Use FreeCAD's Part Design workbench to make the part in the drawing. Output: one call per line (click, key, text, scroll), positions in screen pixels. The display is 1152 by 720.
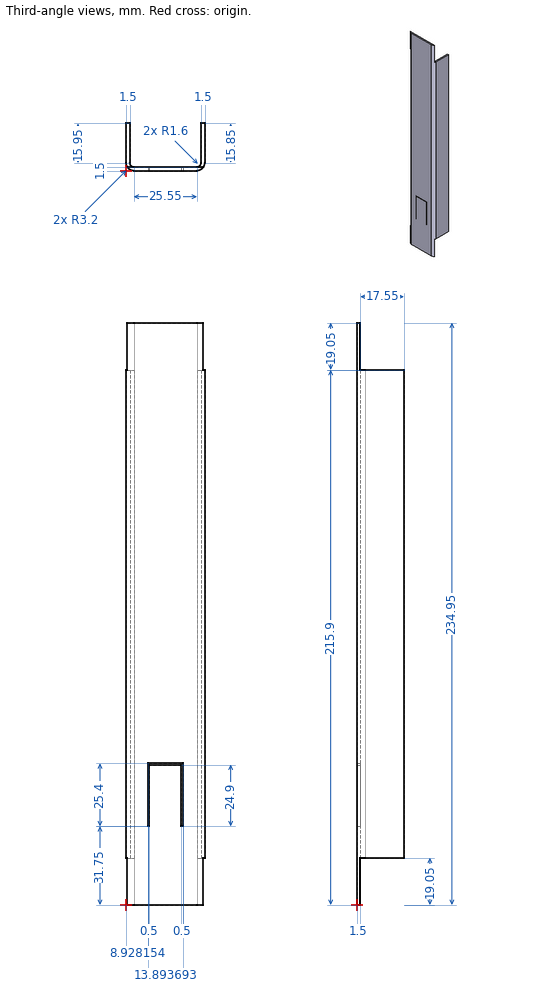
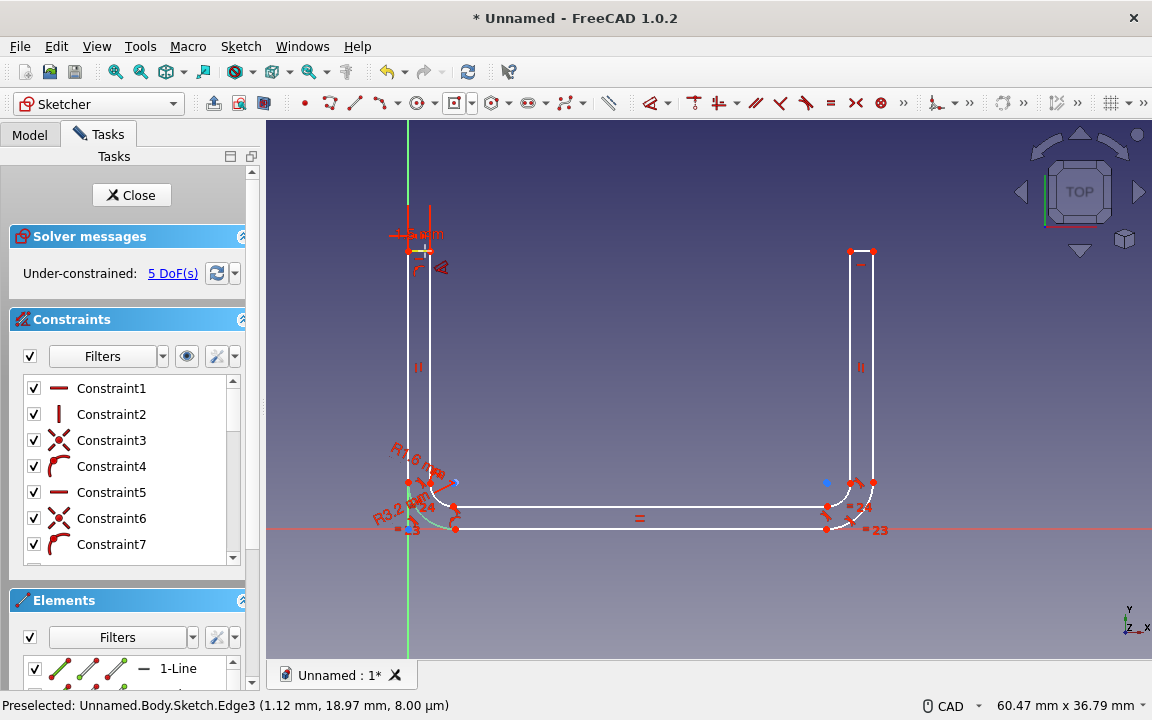
scroll(866, 251, up, 4)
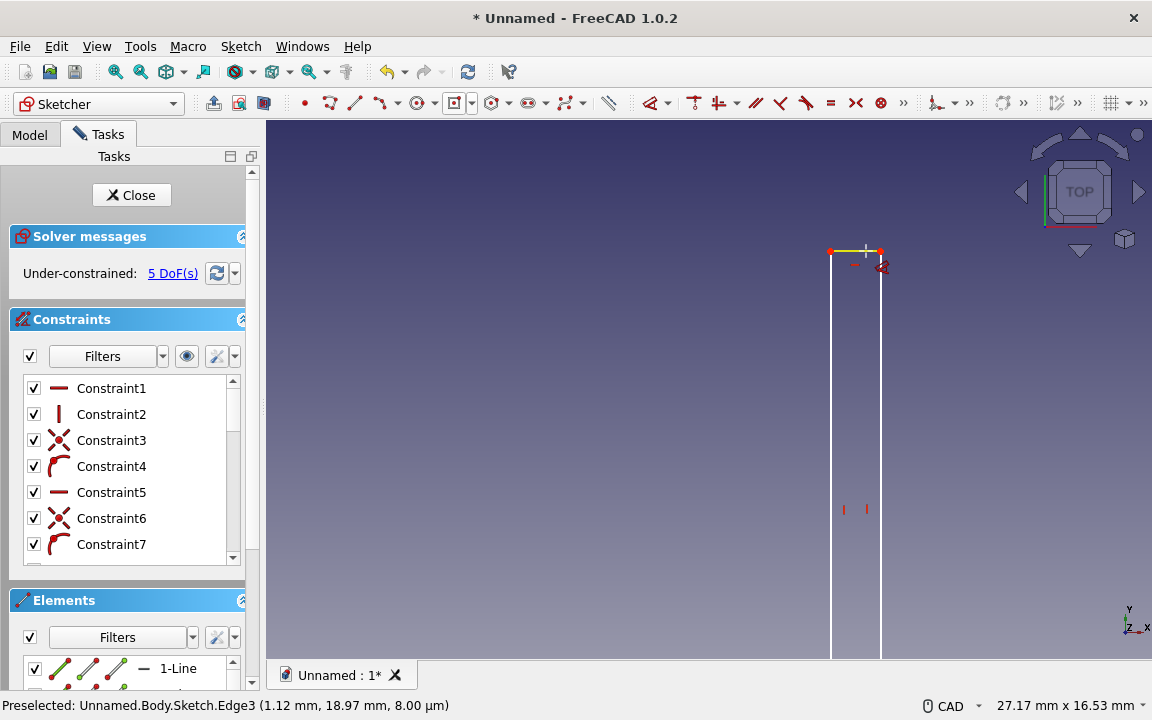
click(866, 251)
click(856, 217)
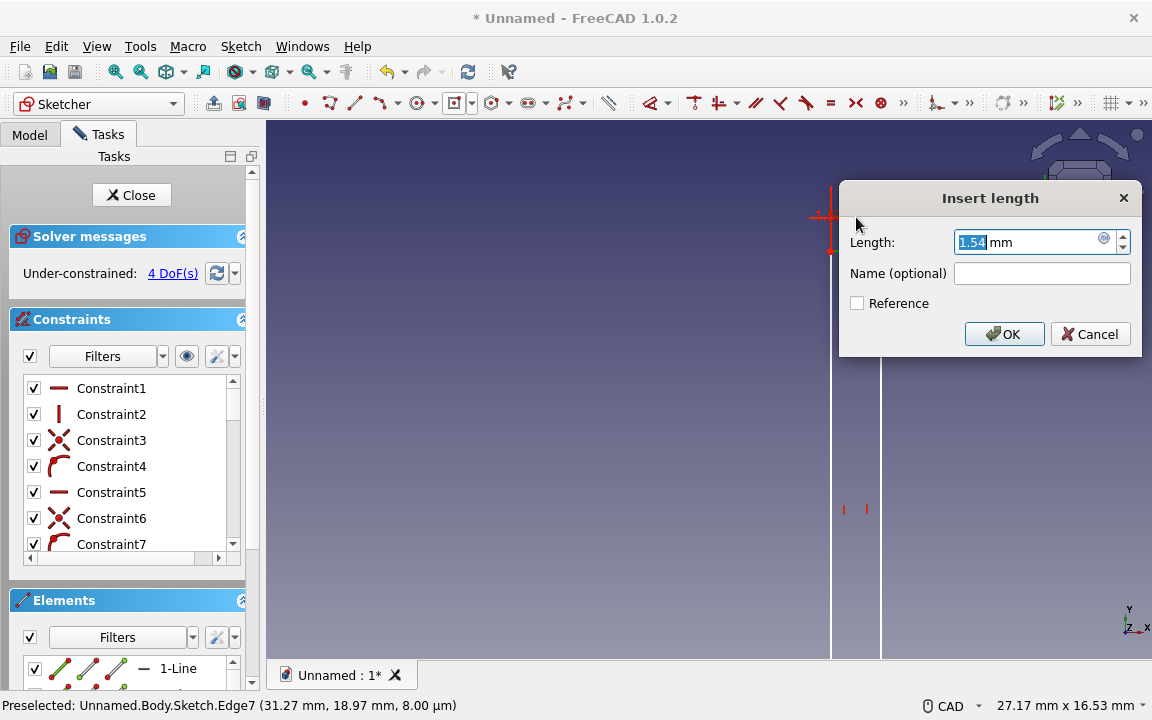
text(1.5)
key(Return)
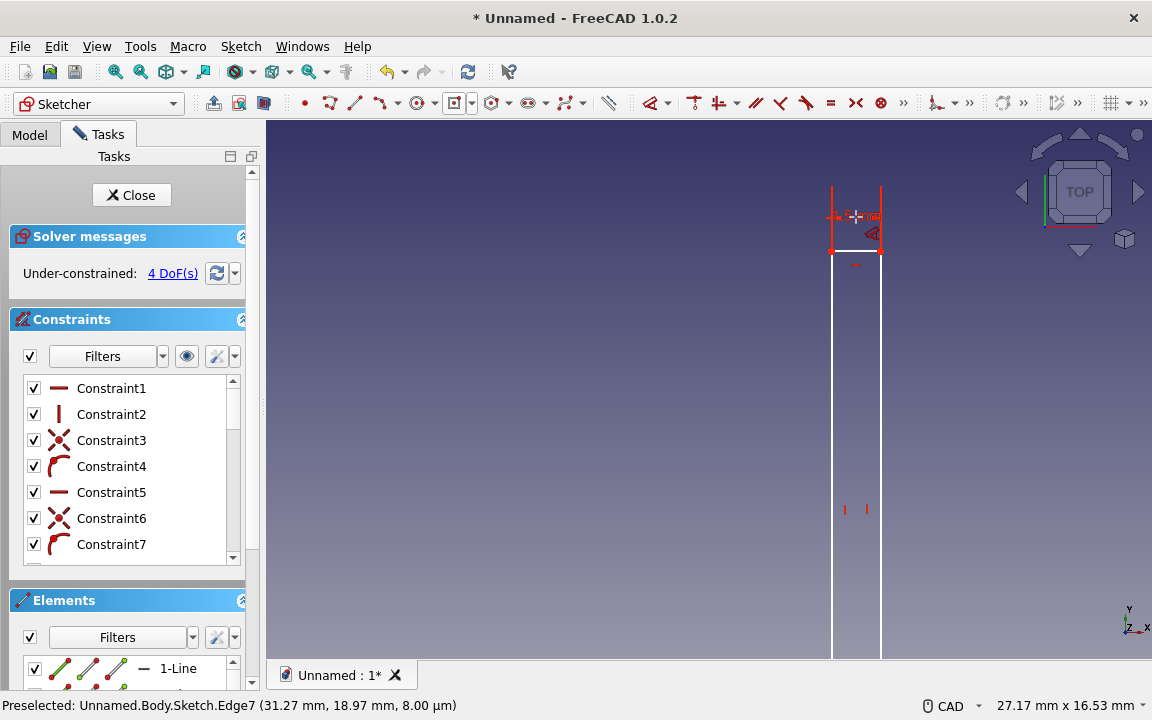
scroll(866, 251, down, 4)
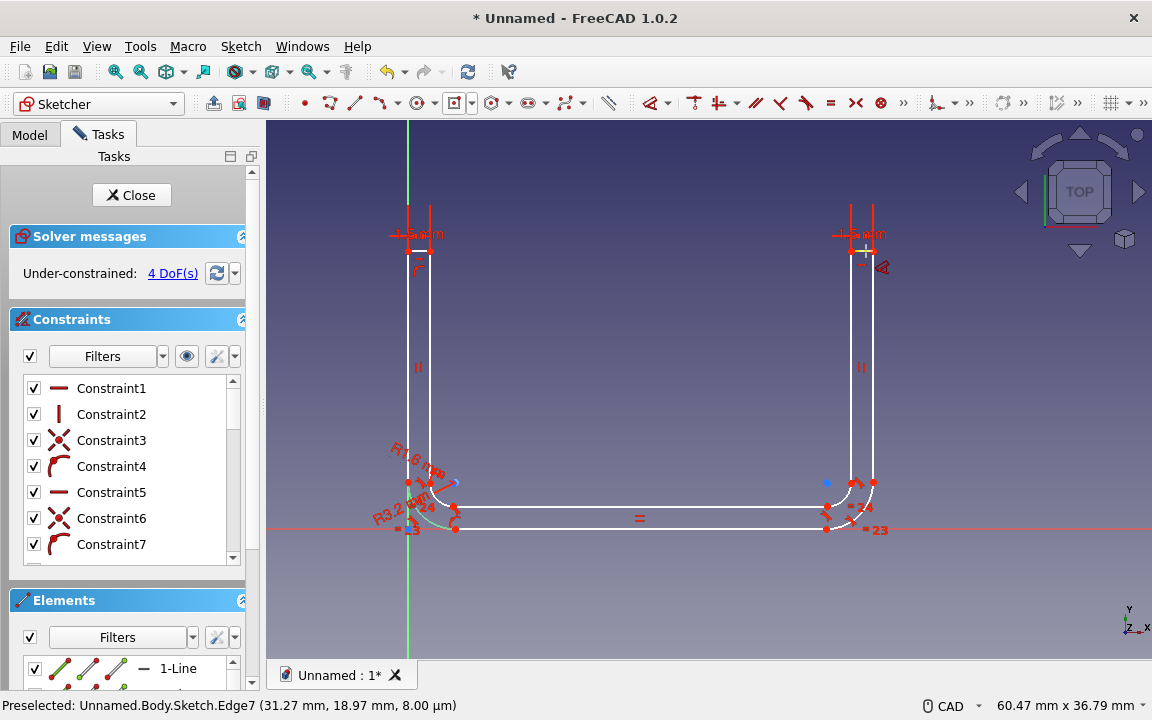
scroll(828, 507, up, 3)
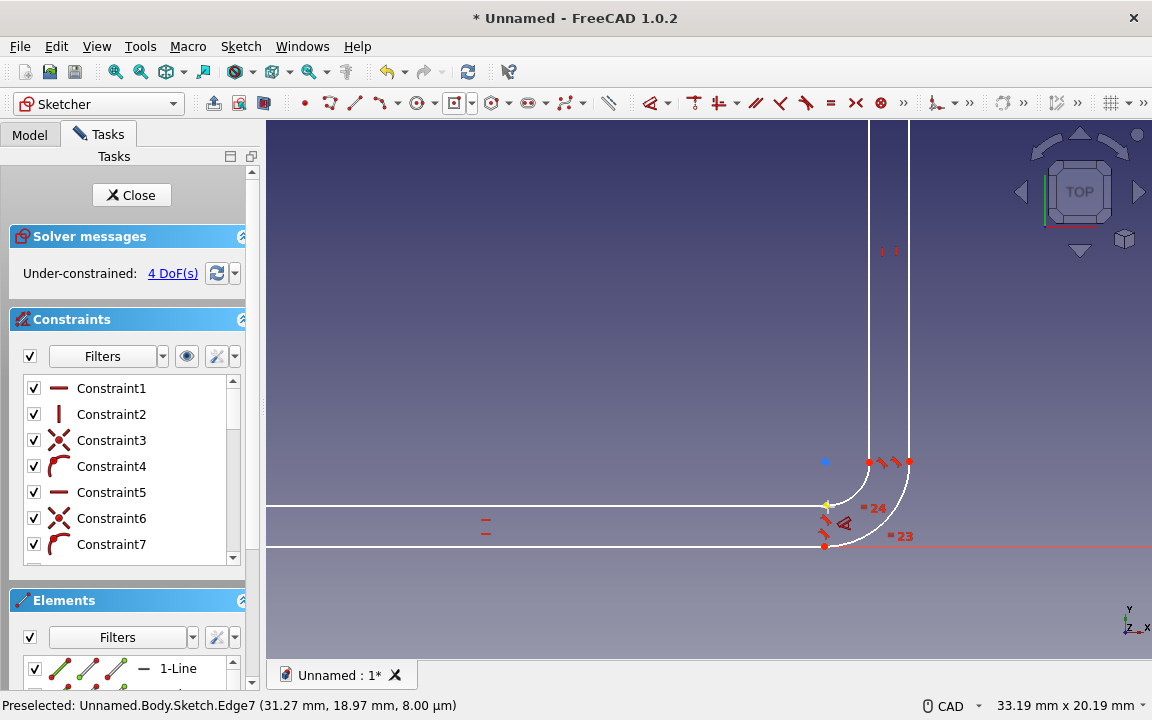
click(827, 506)
click(861, 517)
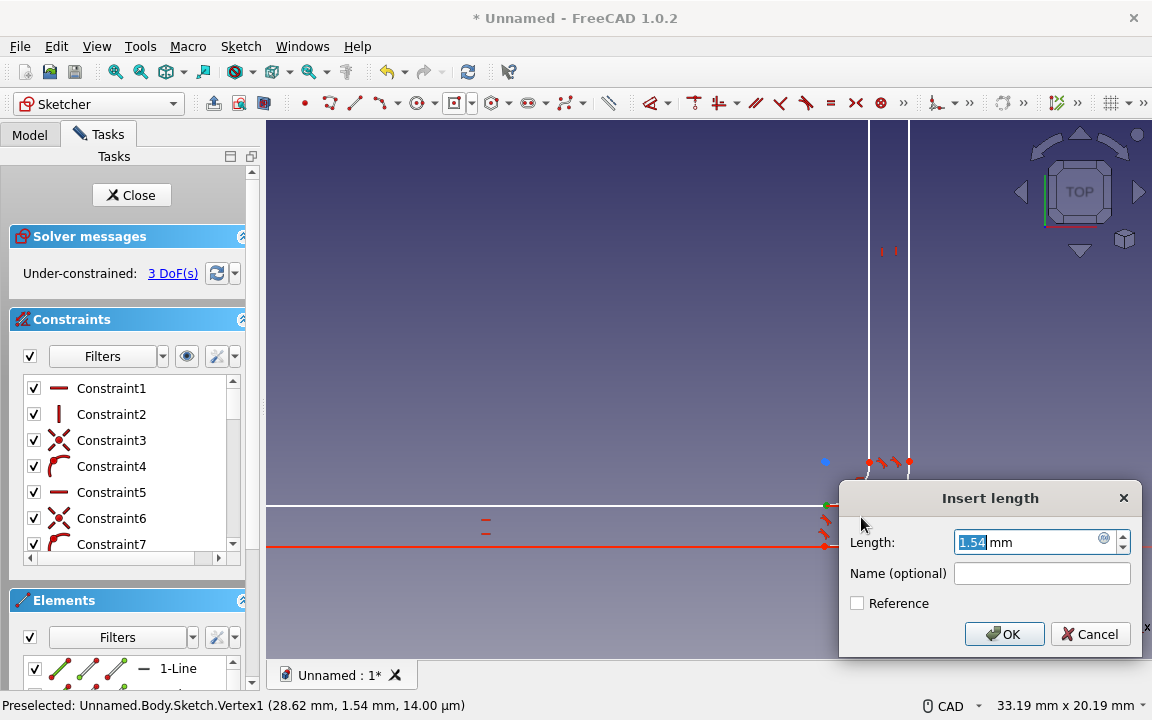
text(1.5)
key(Return)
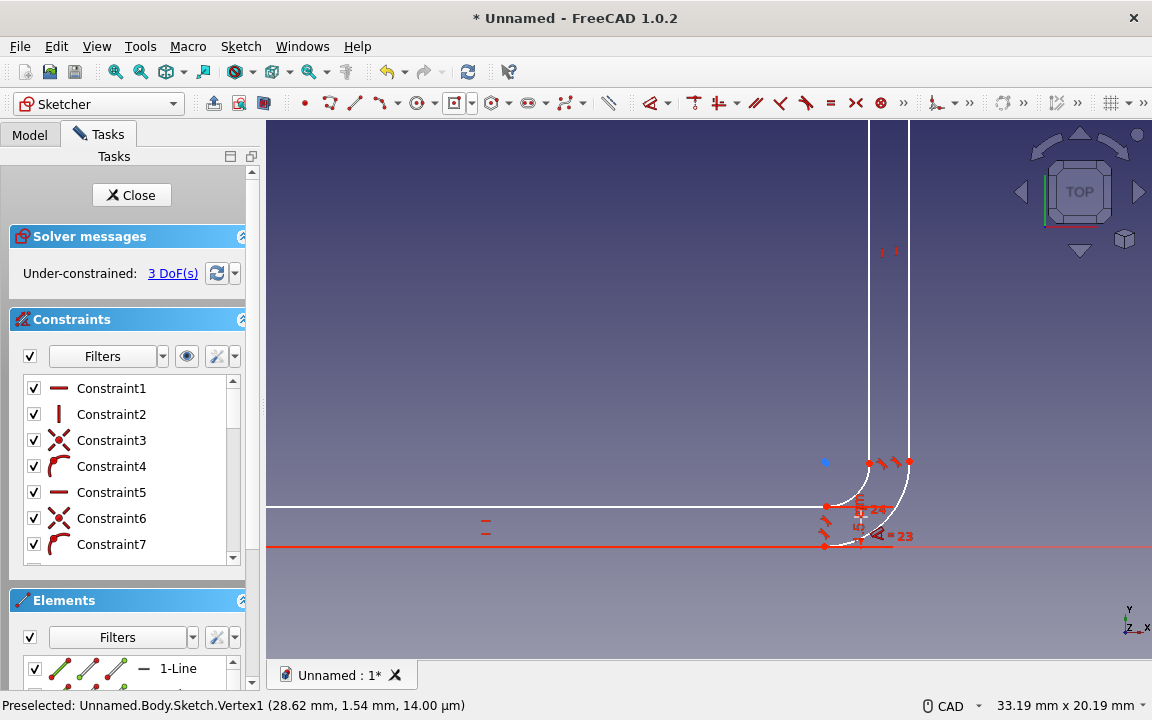
click(622, 507)
click(560, 473)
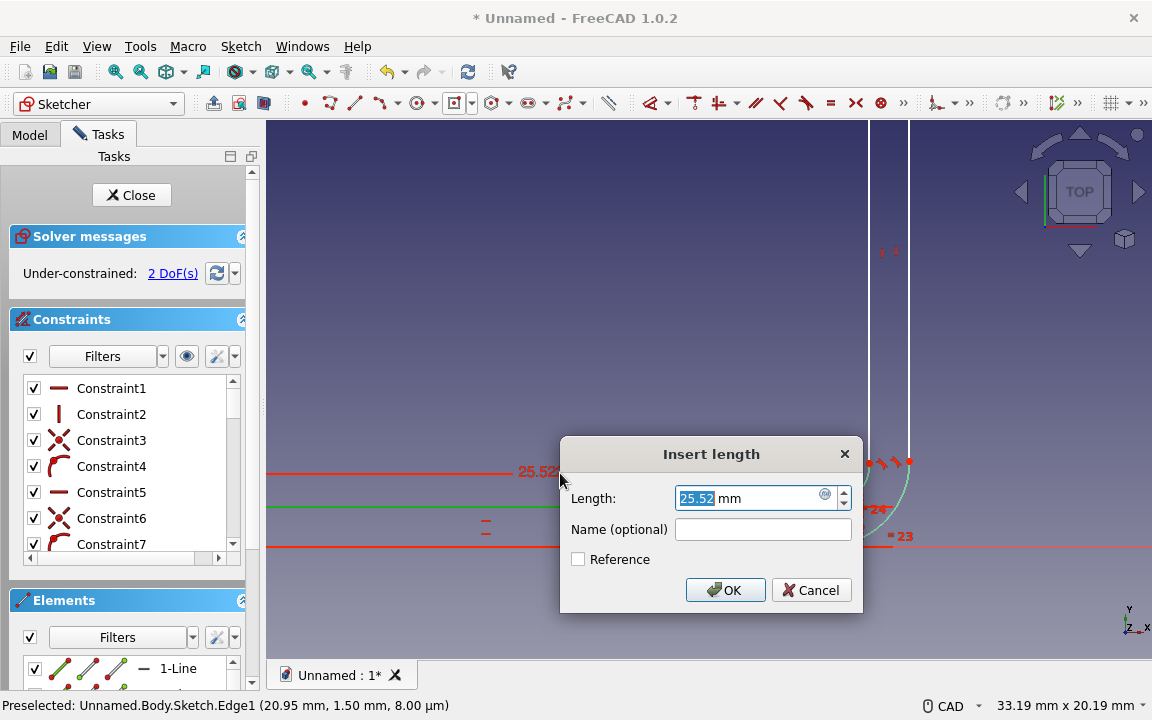
text(25.55)
key(Return)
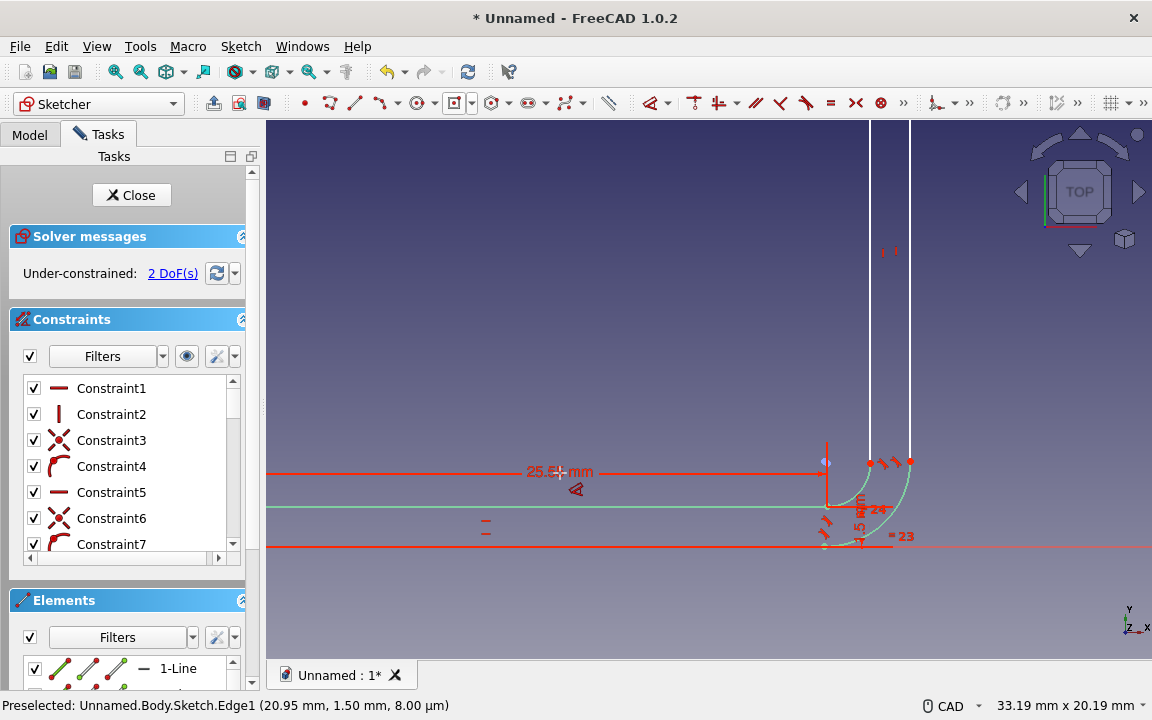
scroll(828, 508, down, 3)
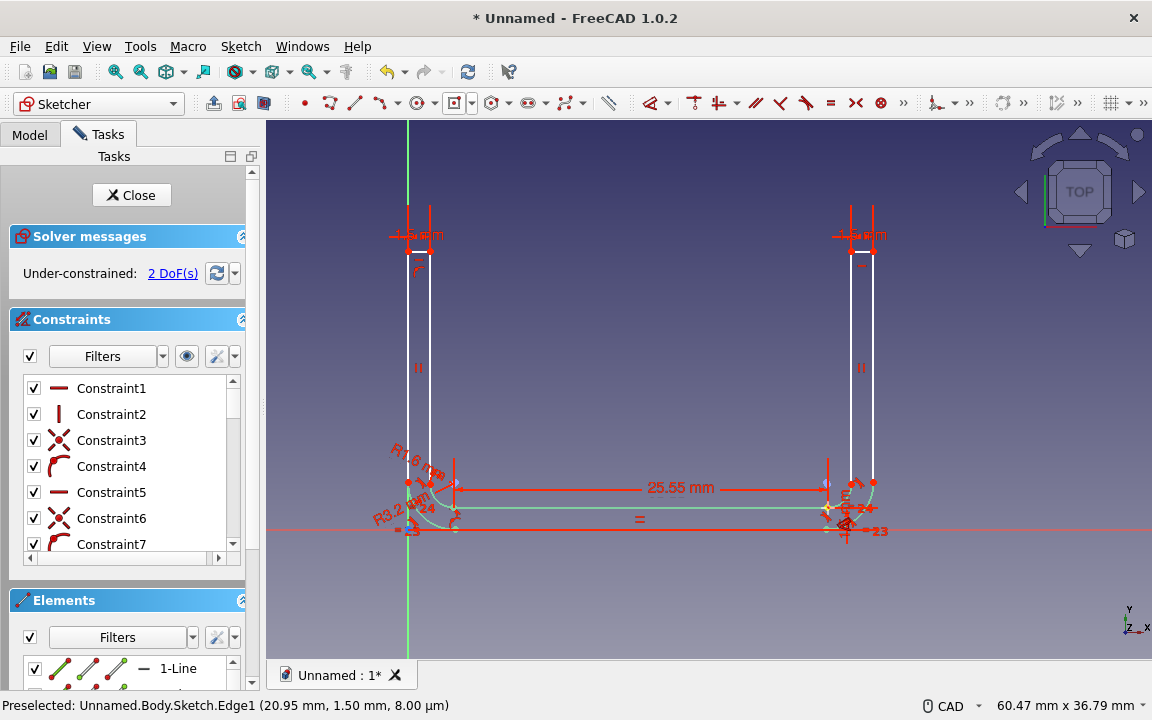
click(430, 414)
click(464, 368)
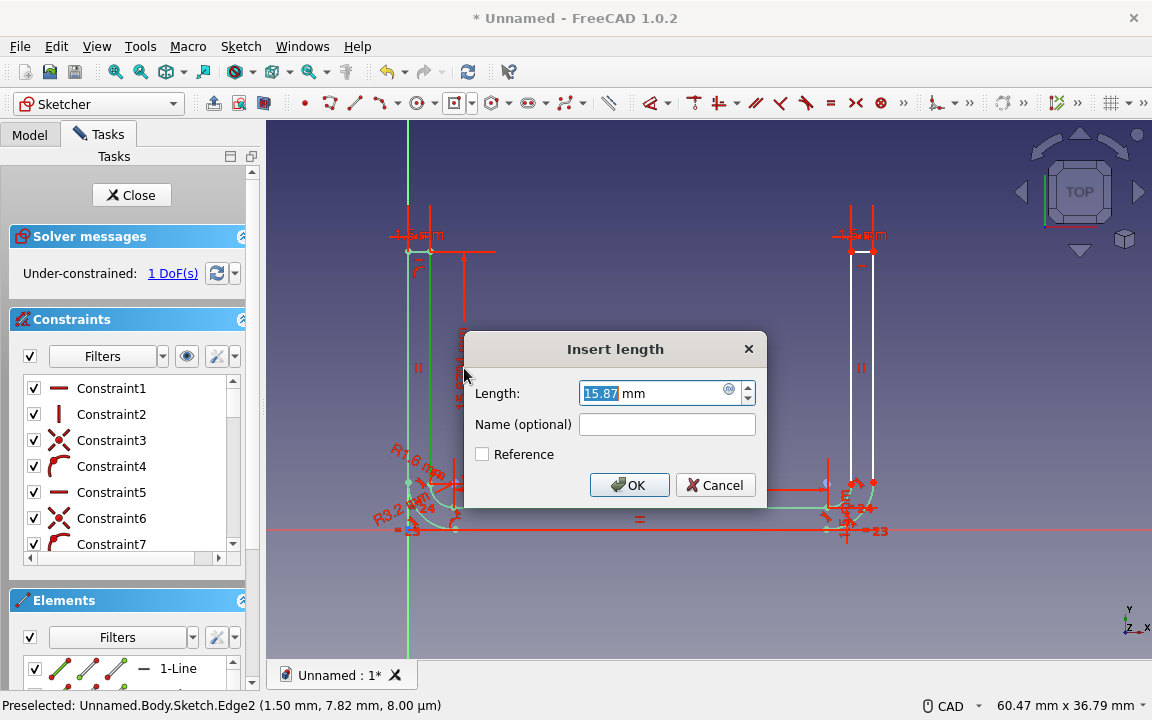
text(15.95)
key(Return)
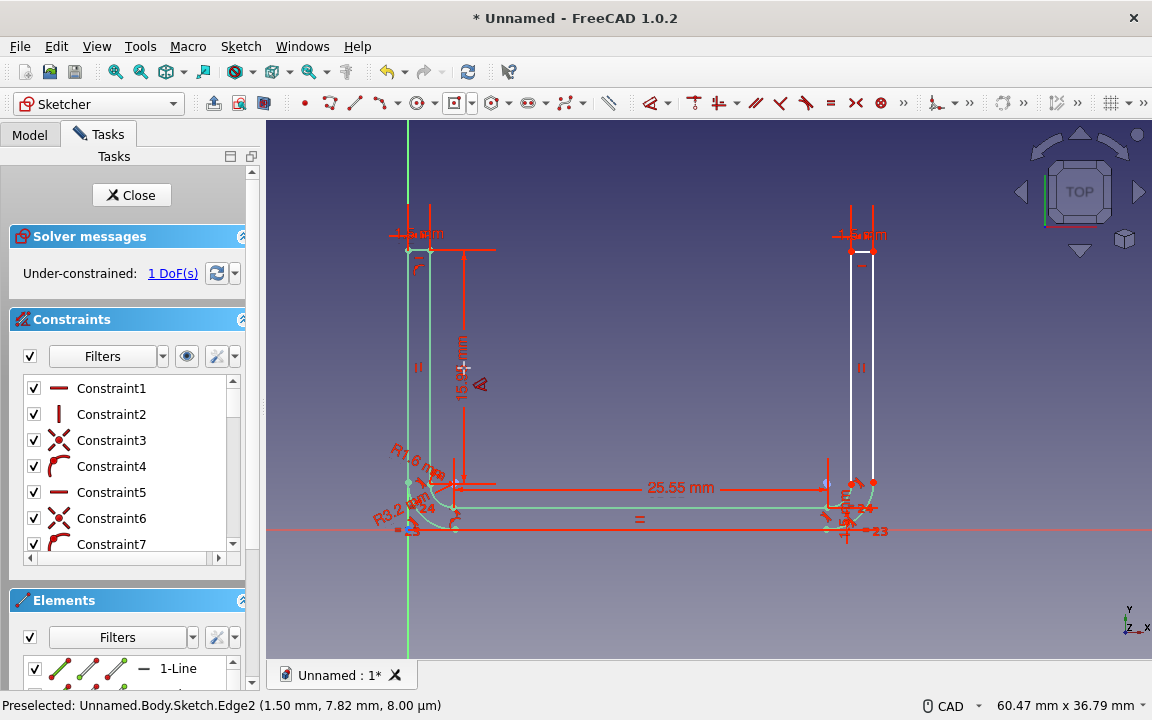
click(873, 413)
click(907, 367)